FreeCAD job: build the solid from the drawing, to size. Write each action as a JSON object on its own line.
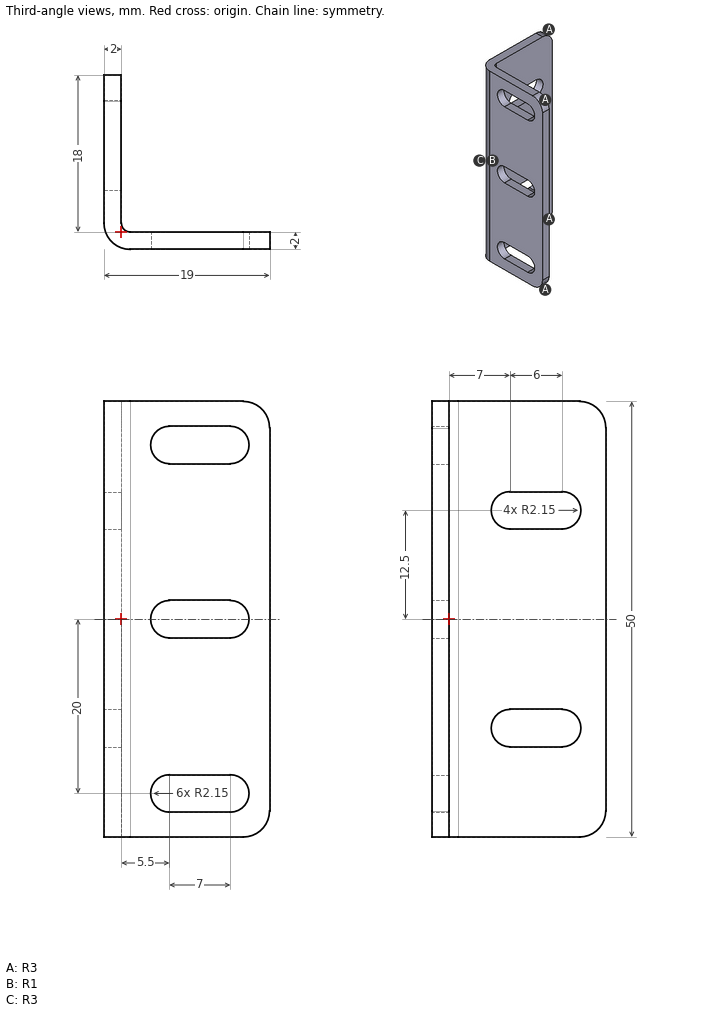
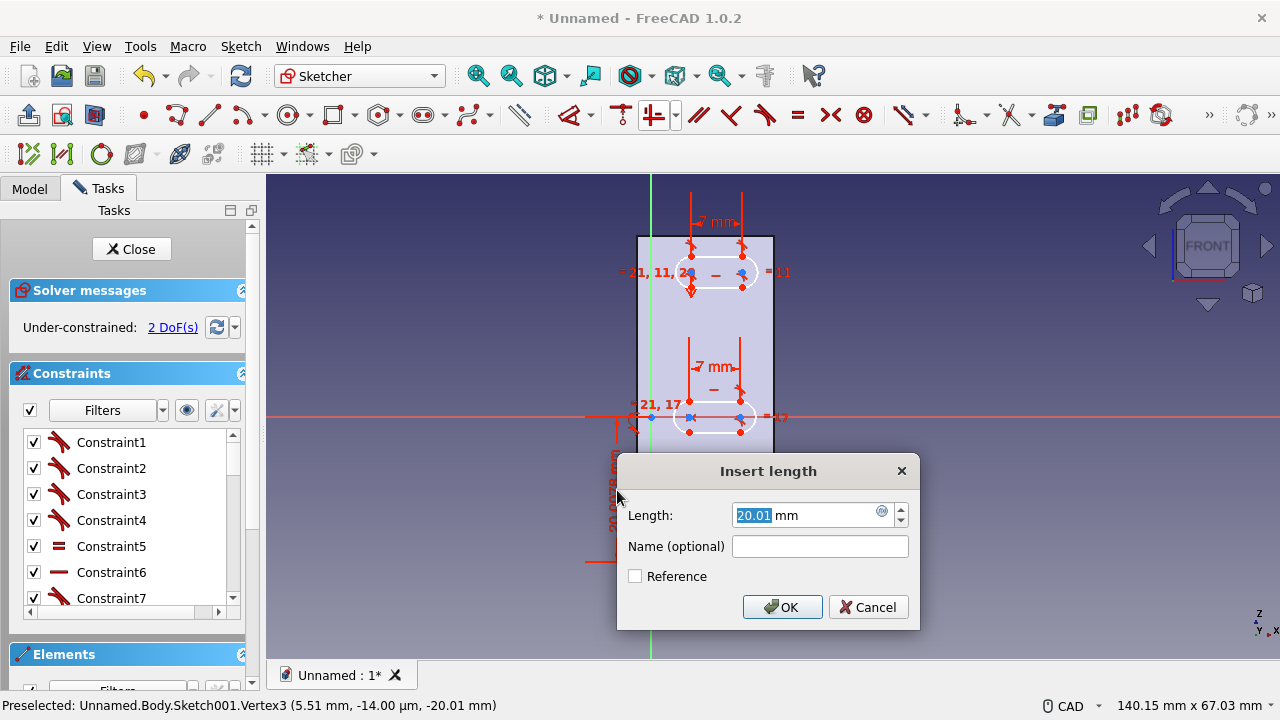
{"action": "type", "text": "20"}
{"action": "key", "text": "Return"}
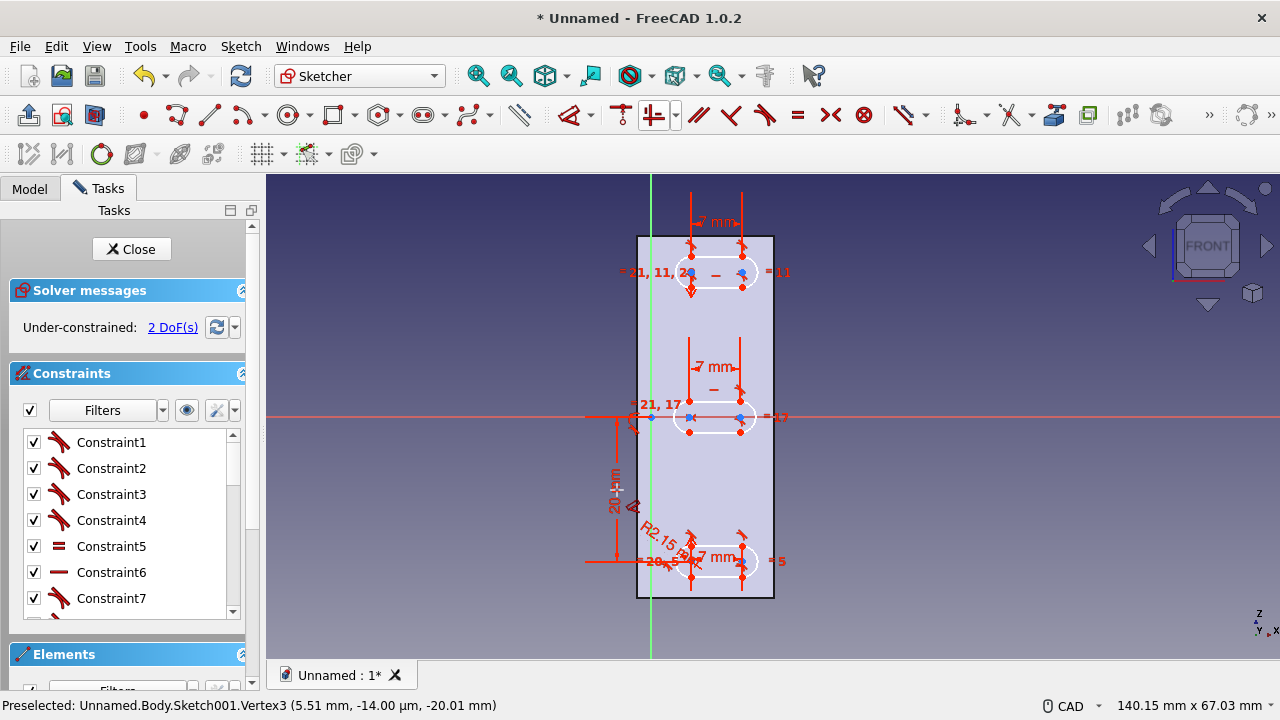
{"action": "left_click", "coordinate": [691, 546]}
{"action": "left_click", "coordinate": [671, 604]}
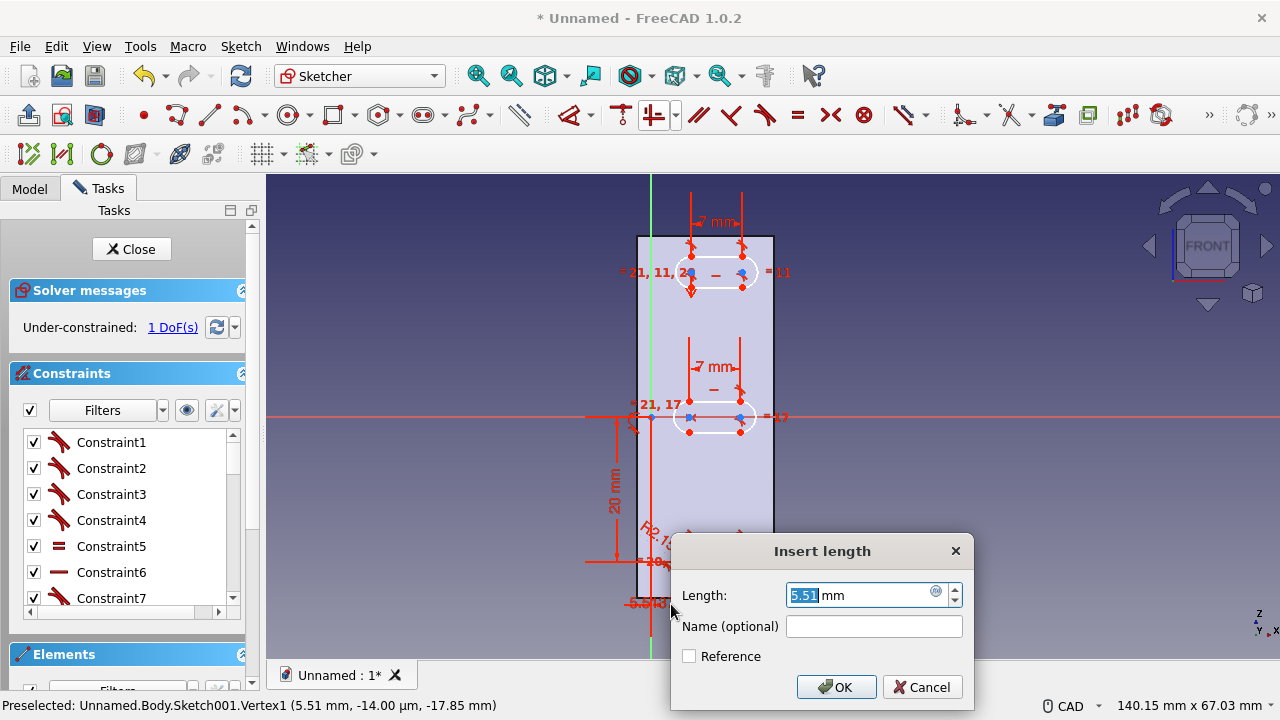
{"action": "type", "text": "5.5"}
{"action": "key", "text": "Return"}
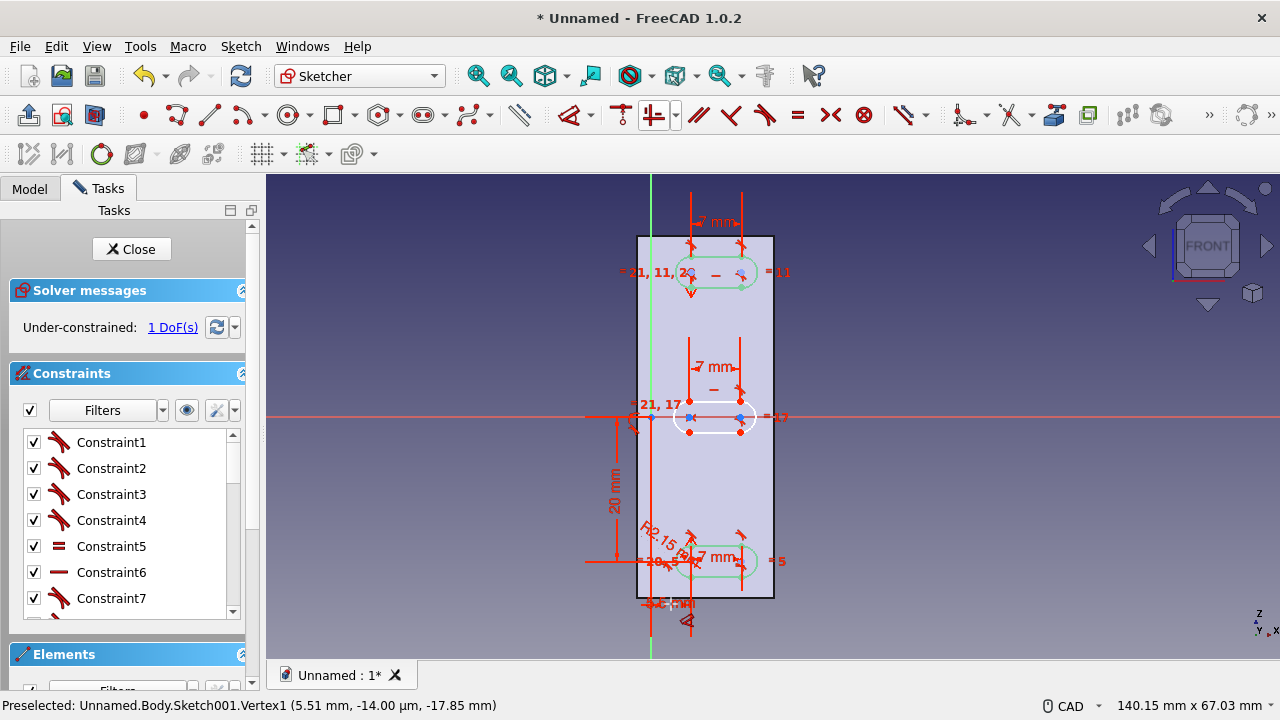
{"action": "left_click", "coordinate": [689, 402]}
{"action": "left_click", "coordinate": [670, 451]}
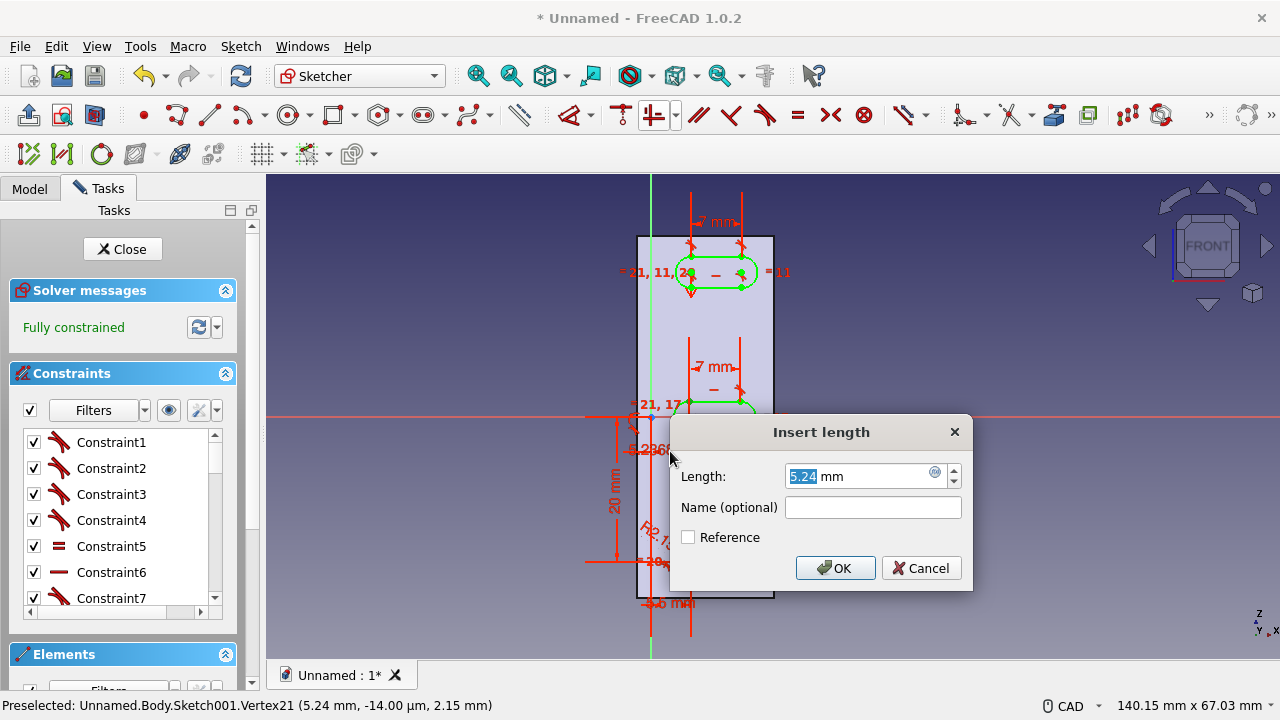
{"action": "type", "text": "5.5"}
{"action": "key", "text": "Return"}
{"action": "key", "text": "Escape"}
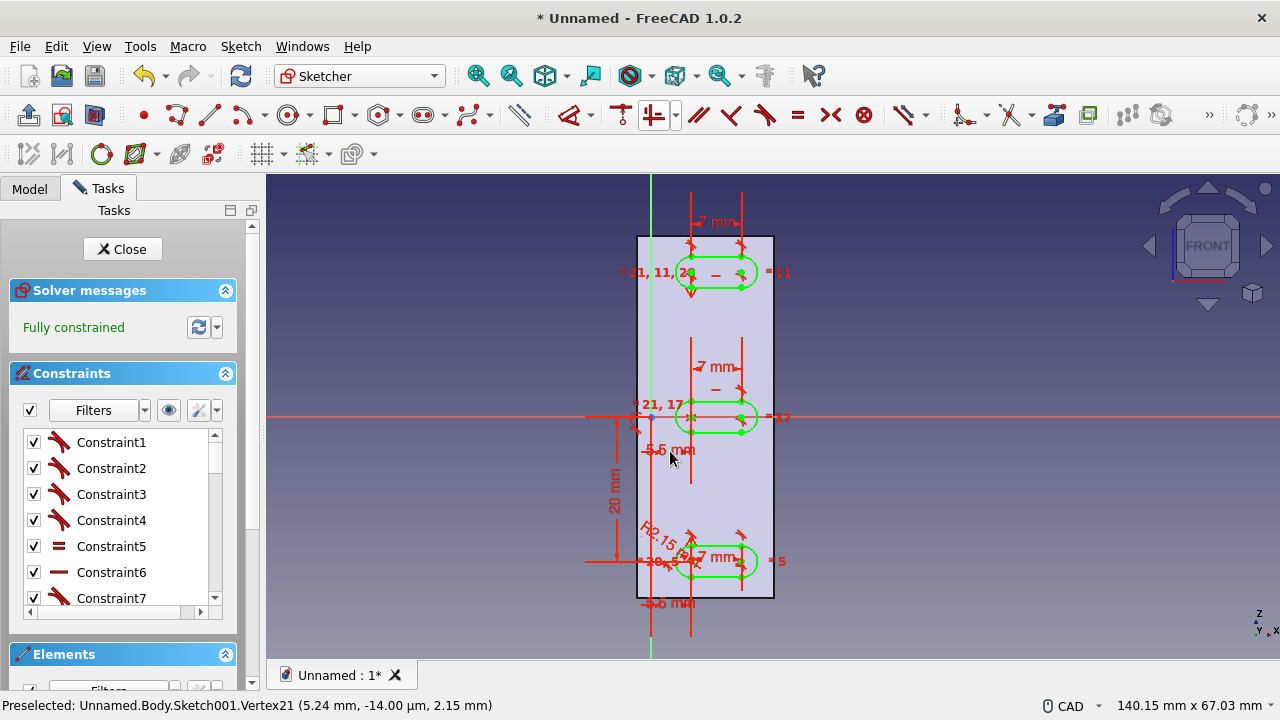
{"action": "left_click", "coordinate": [123, 249]}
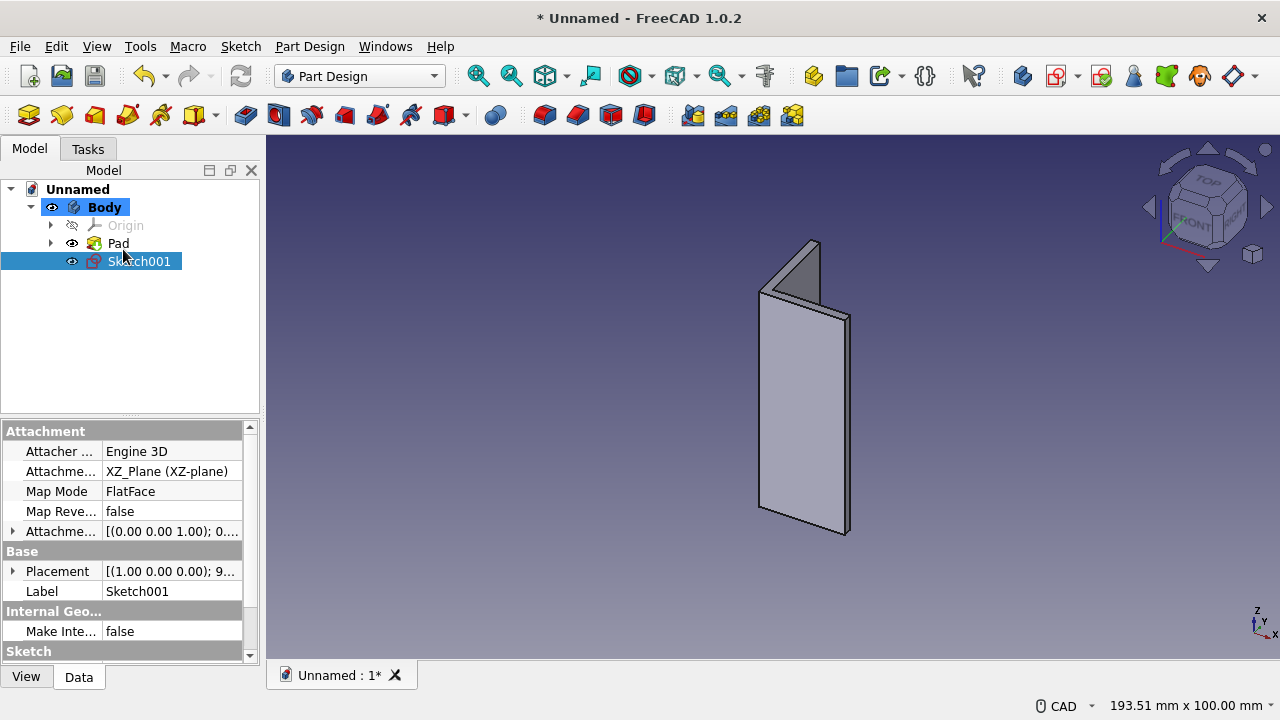
{"action": "left_click", "coordinate": [246, 116]}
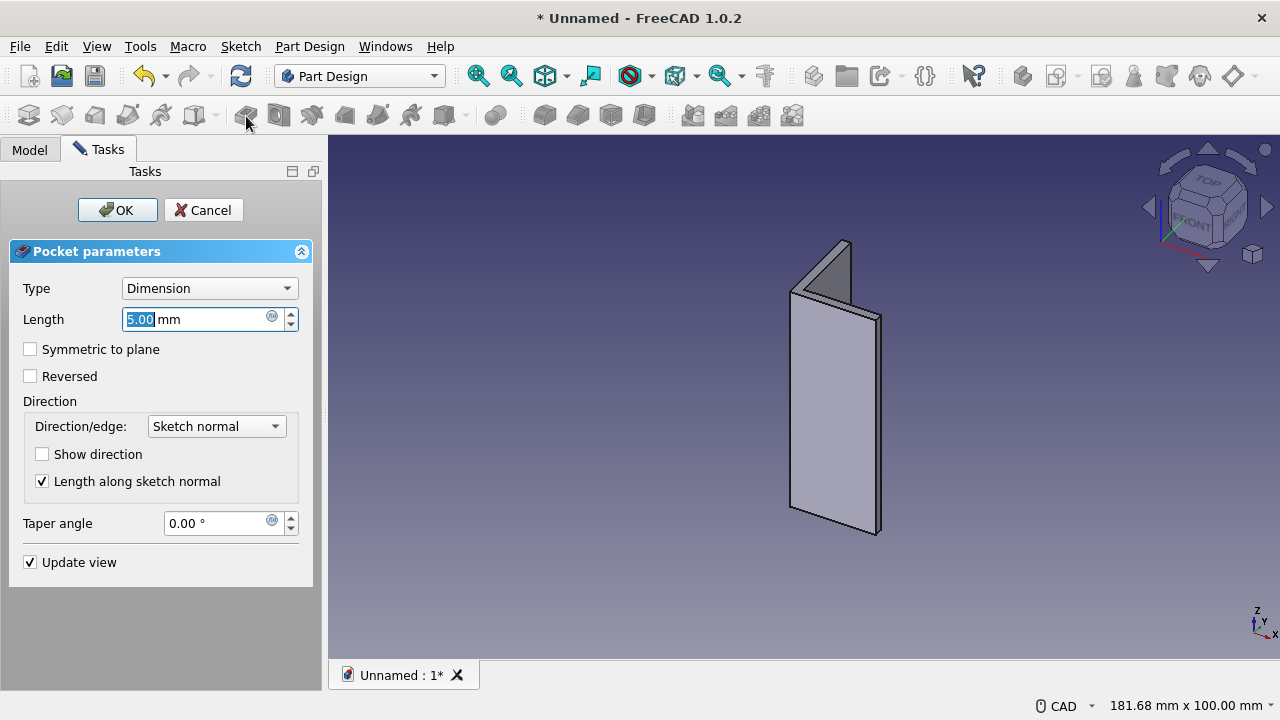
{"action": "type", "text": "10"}
{"action": "key", "text": "Tab"}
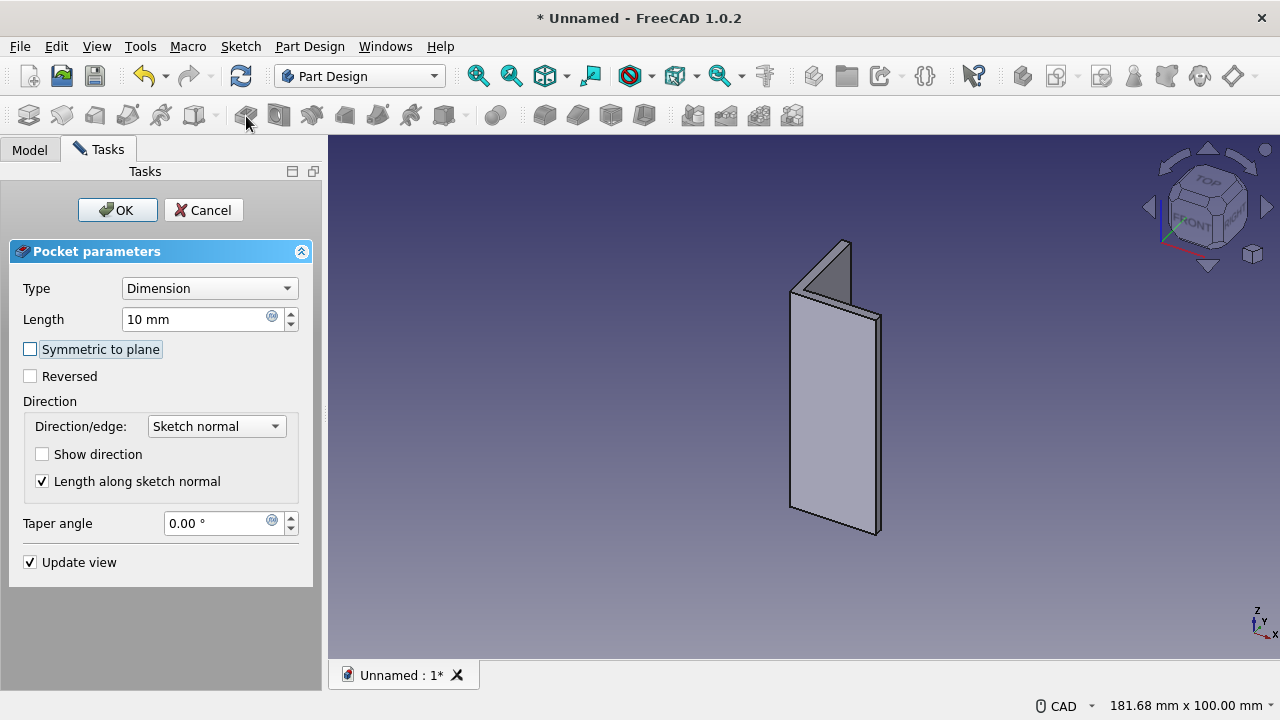
{"action": "left_click", "coordinate": [31, 376]}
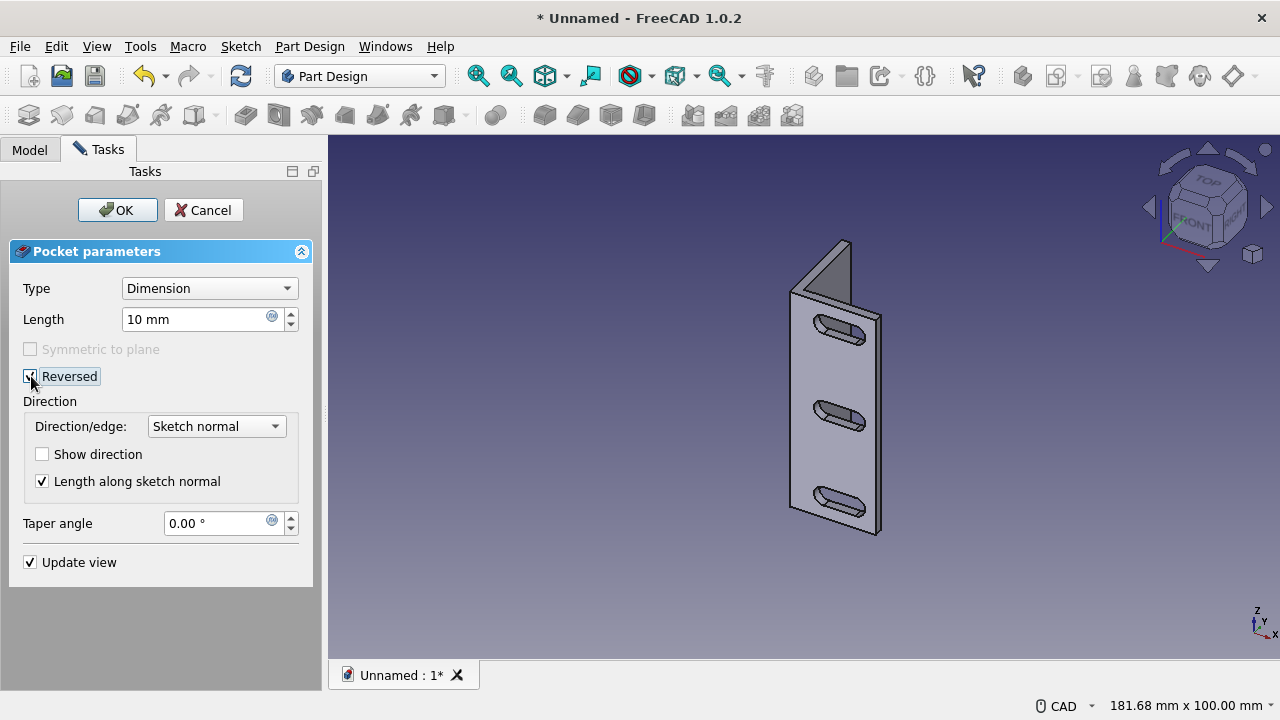
{"action": "left_click", "coordinate": [118, 210]}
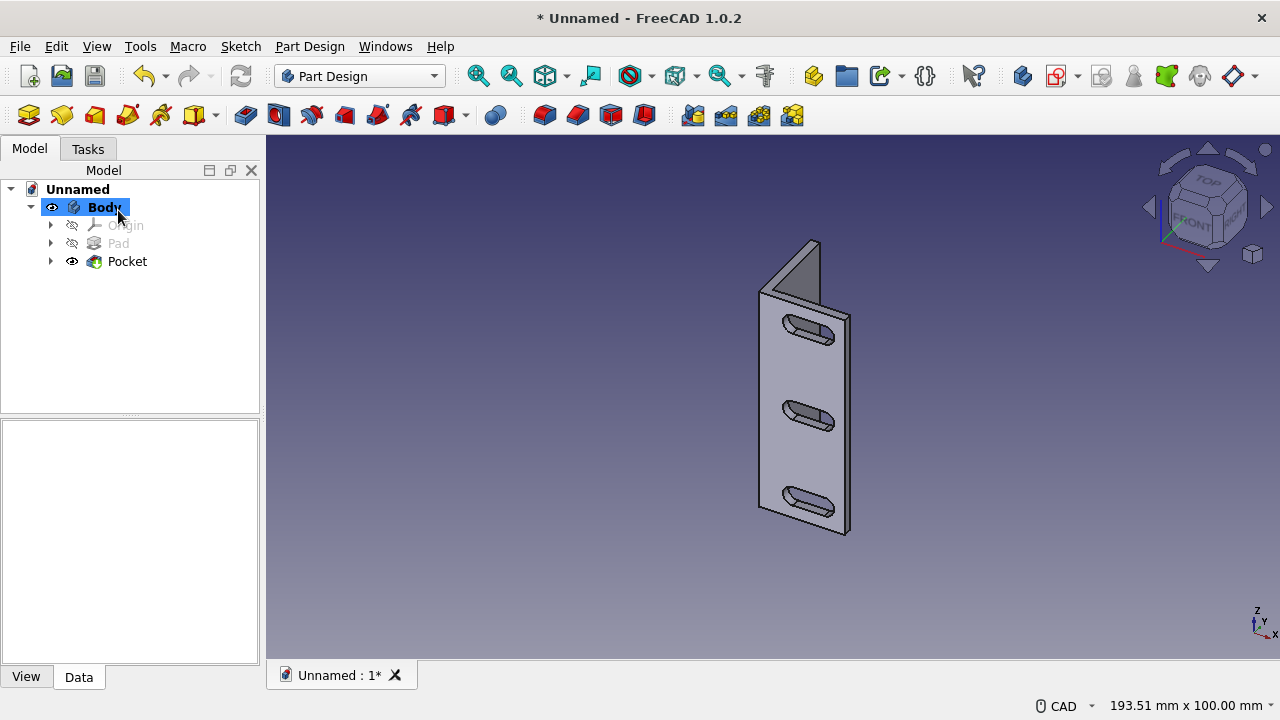
{"action": "left_click", "coordinate": [1056, 76]}